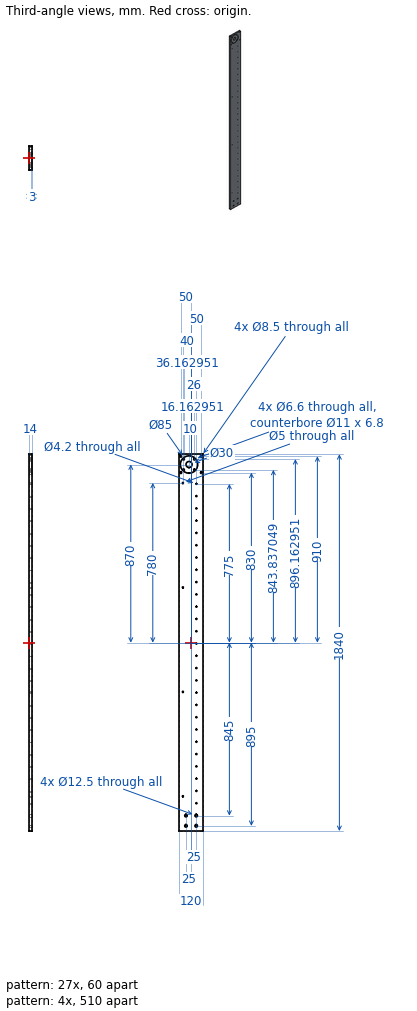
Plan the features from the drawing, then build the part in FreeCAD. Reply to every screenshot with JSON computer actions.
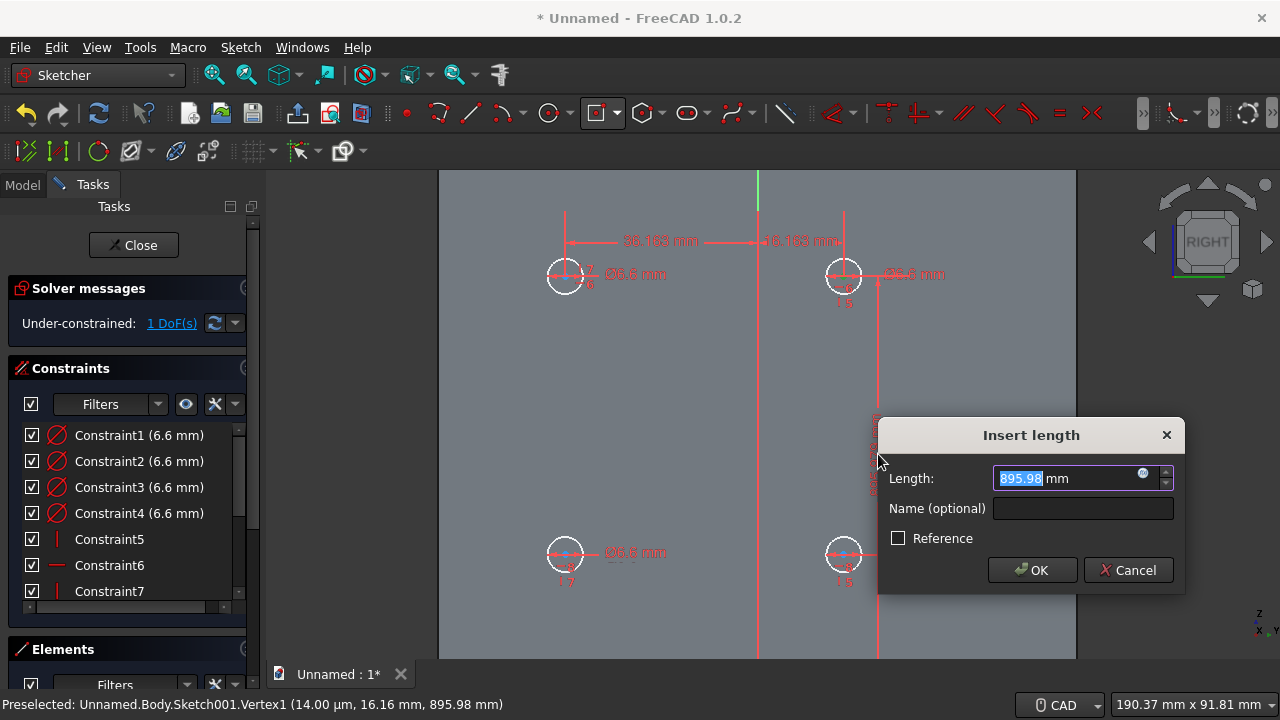
{"action": "type", "text": "896.162951"}
{"action": "key", "text": "Return"}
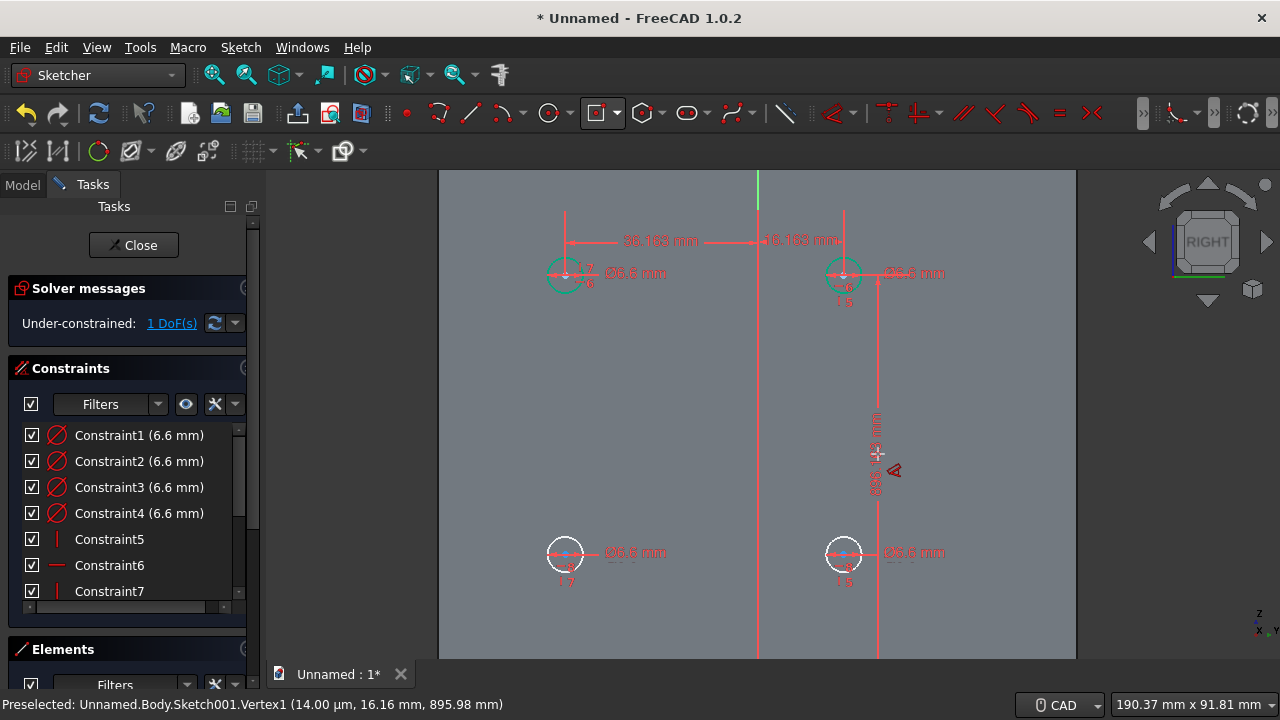
{"action": "left_click", "coordinate": [844, 555]}
{"action": "left_click", "coordinate": [878, 593]}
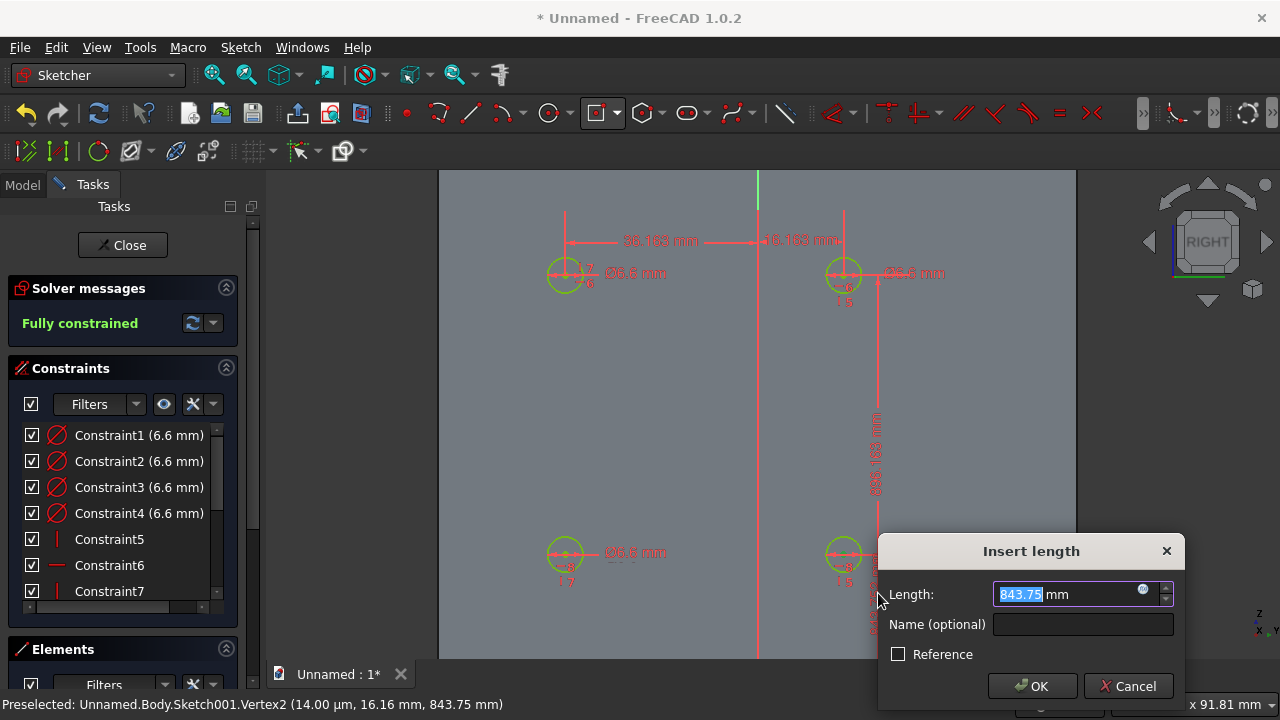
{"action": "type", "text": "843.837049"}
{"action": "key", "text": "Return"}
{"action": "key", "text": "Escape"}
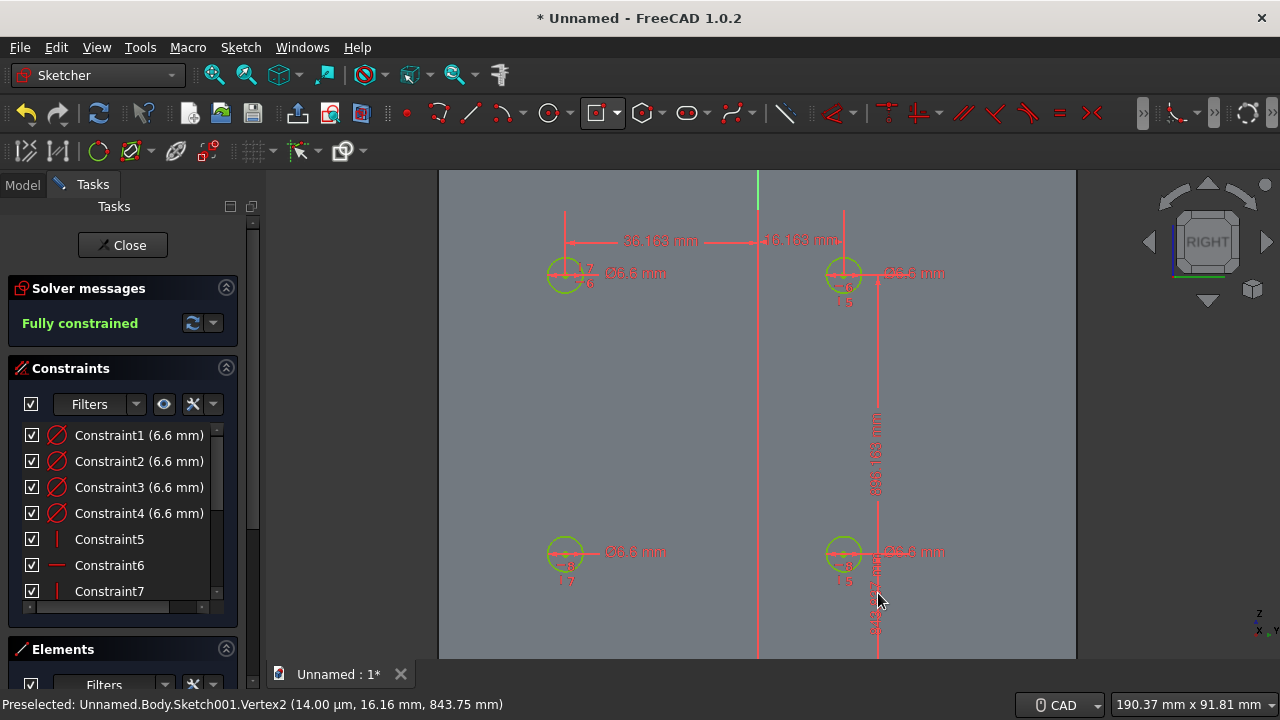
{"action": "left_click", "coordinate": [123, 245]}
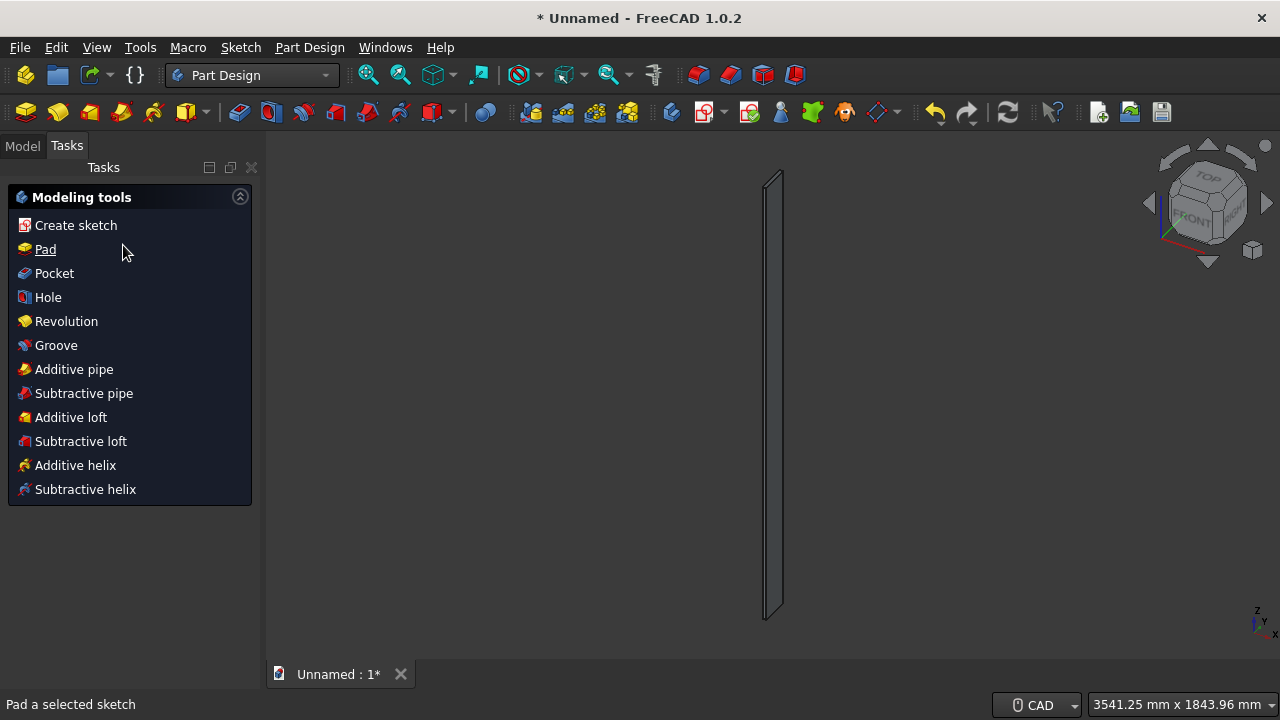
{"action": "left_click", "coordinate": [272, 112]}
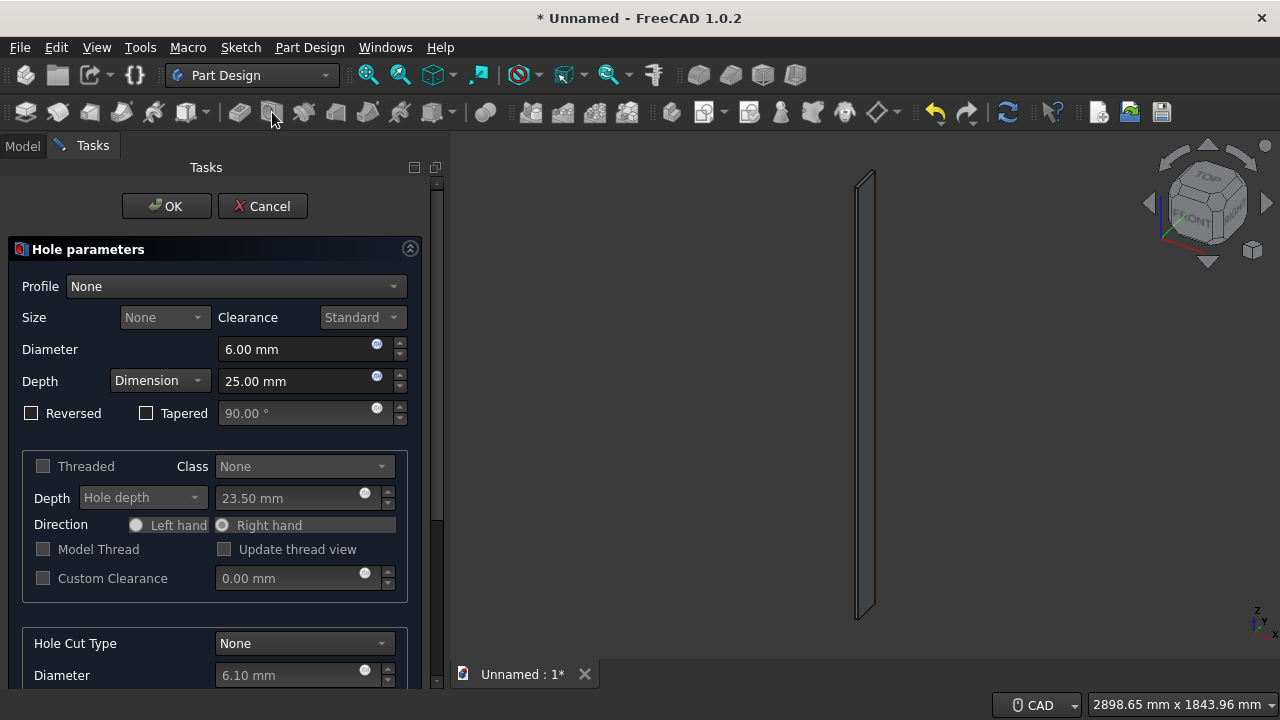
{"action": "triple_click", "coordinate": [305, 349]}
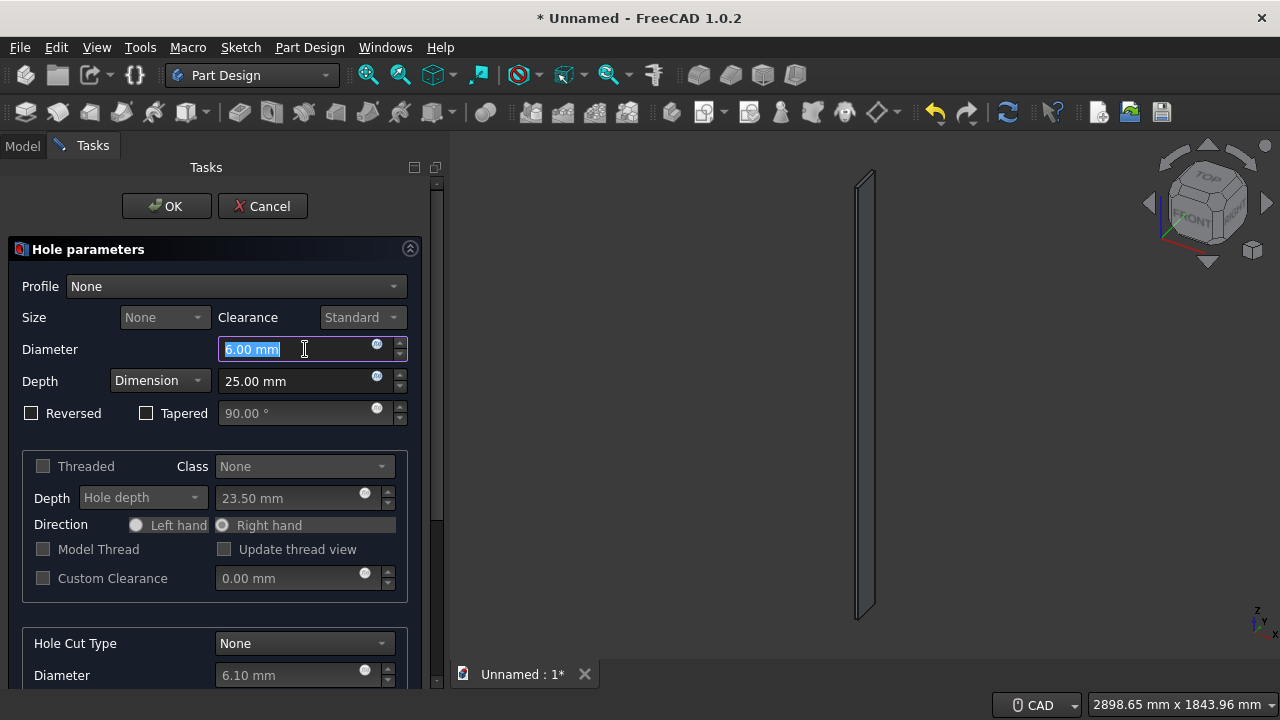
{"action": "type", "text": "6.6"}
{"action": "key", "text": "Tab"}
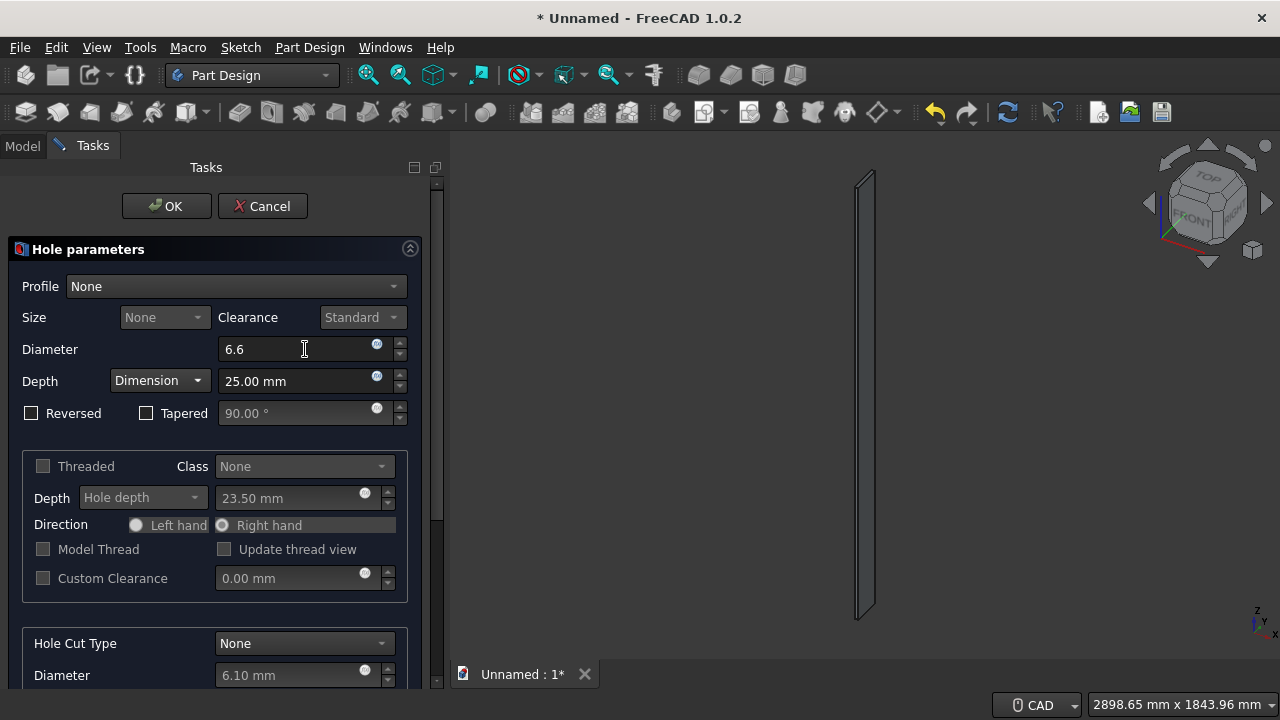
{"action": "left_click", "coordinate": [161, 380]}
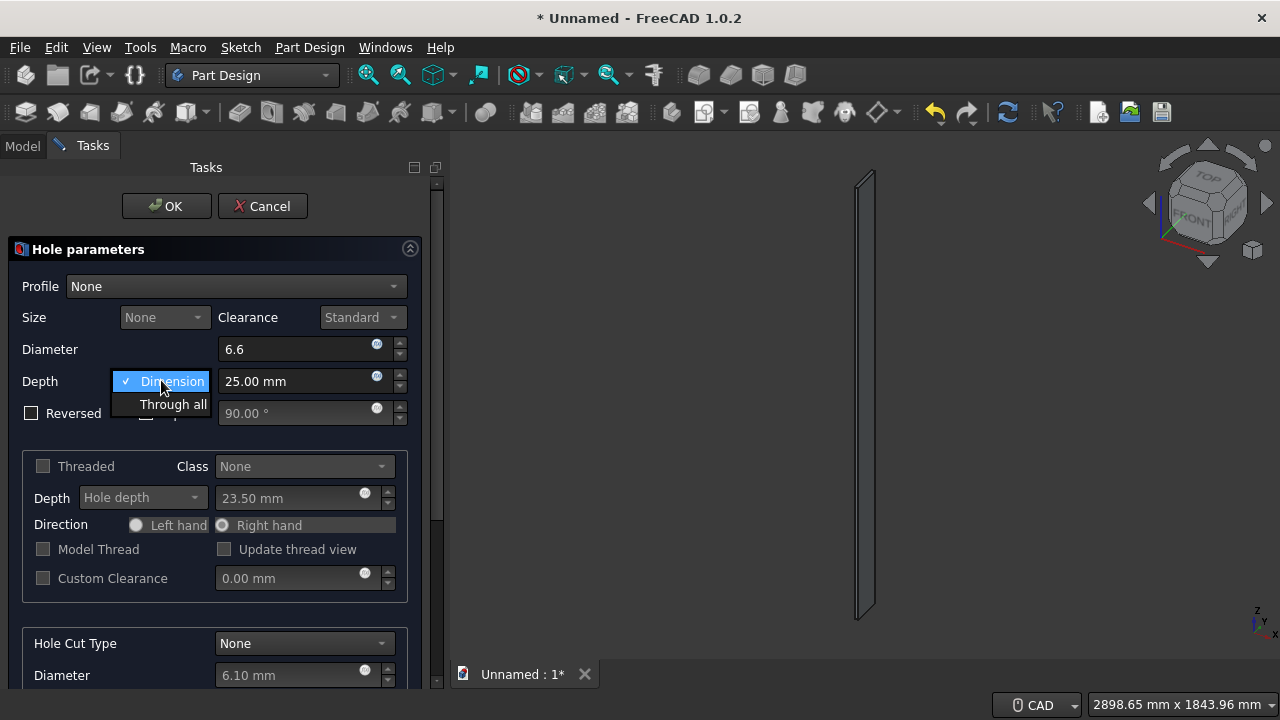
{"action": "left_click", "coordinate": [160, 404]}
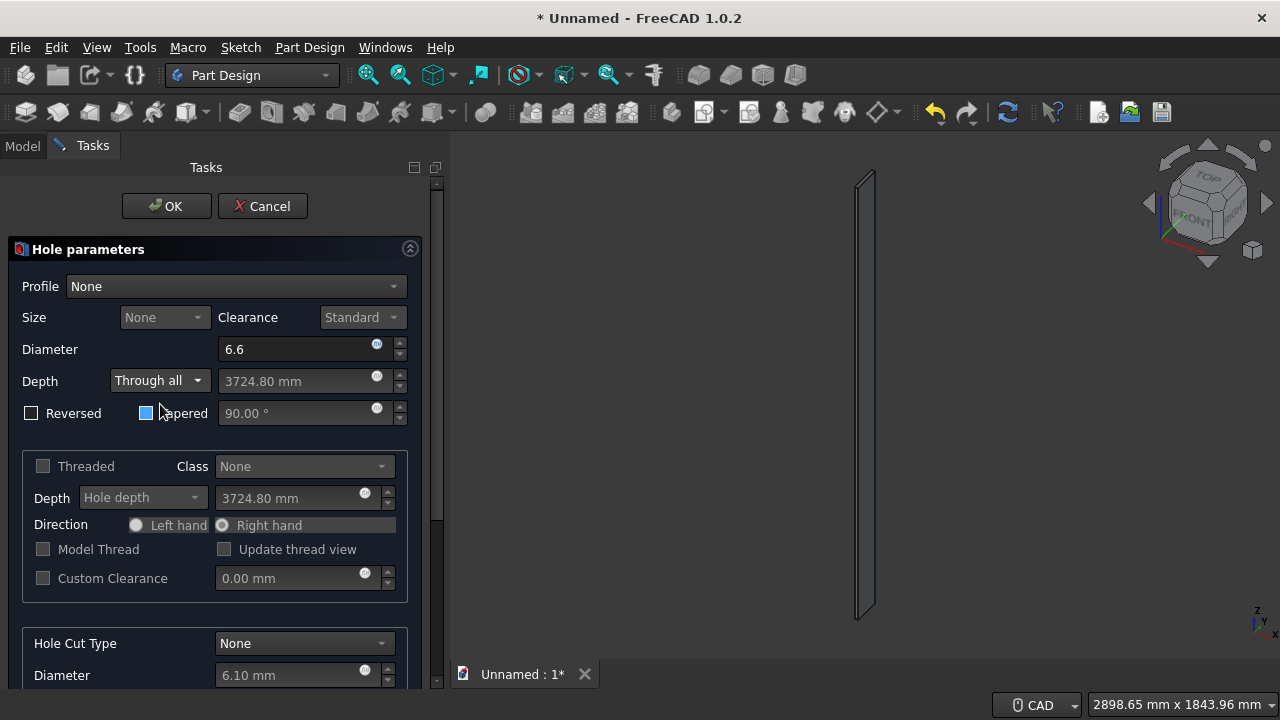
{"action": "left_click", "coordinate": [30, 413]}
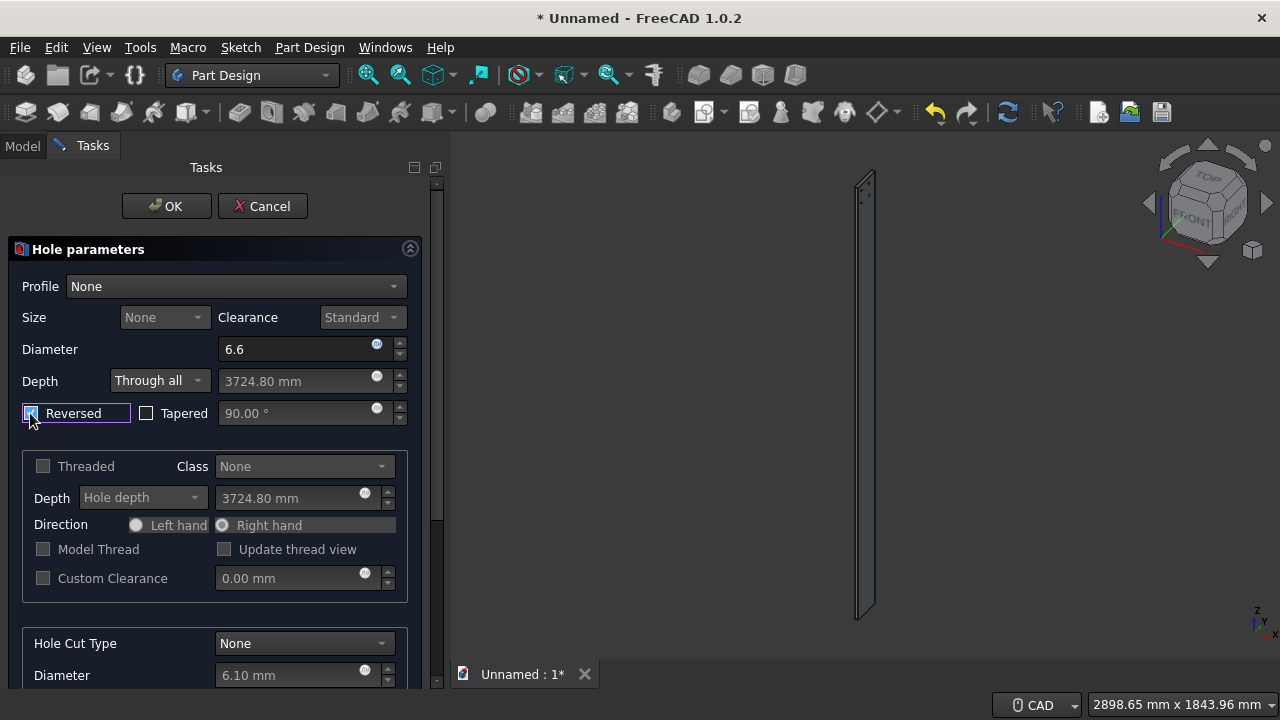
{"action": "left_click", "coordinate": [306, 644]}